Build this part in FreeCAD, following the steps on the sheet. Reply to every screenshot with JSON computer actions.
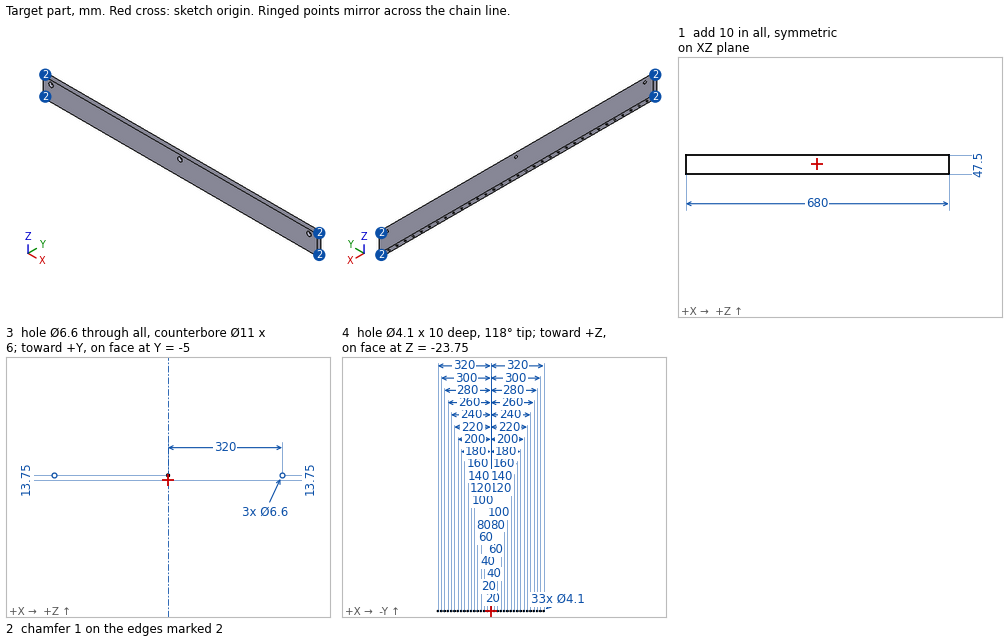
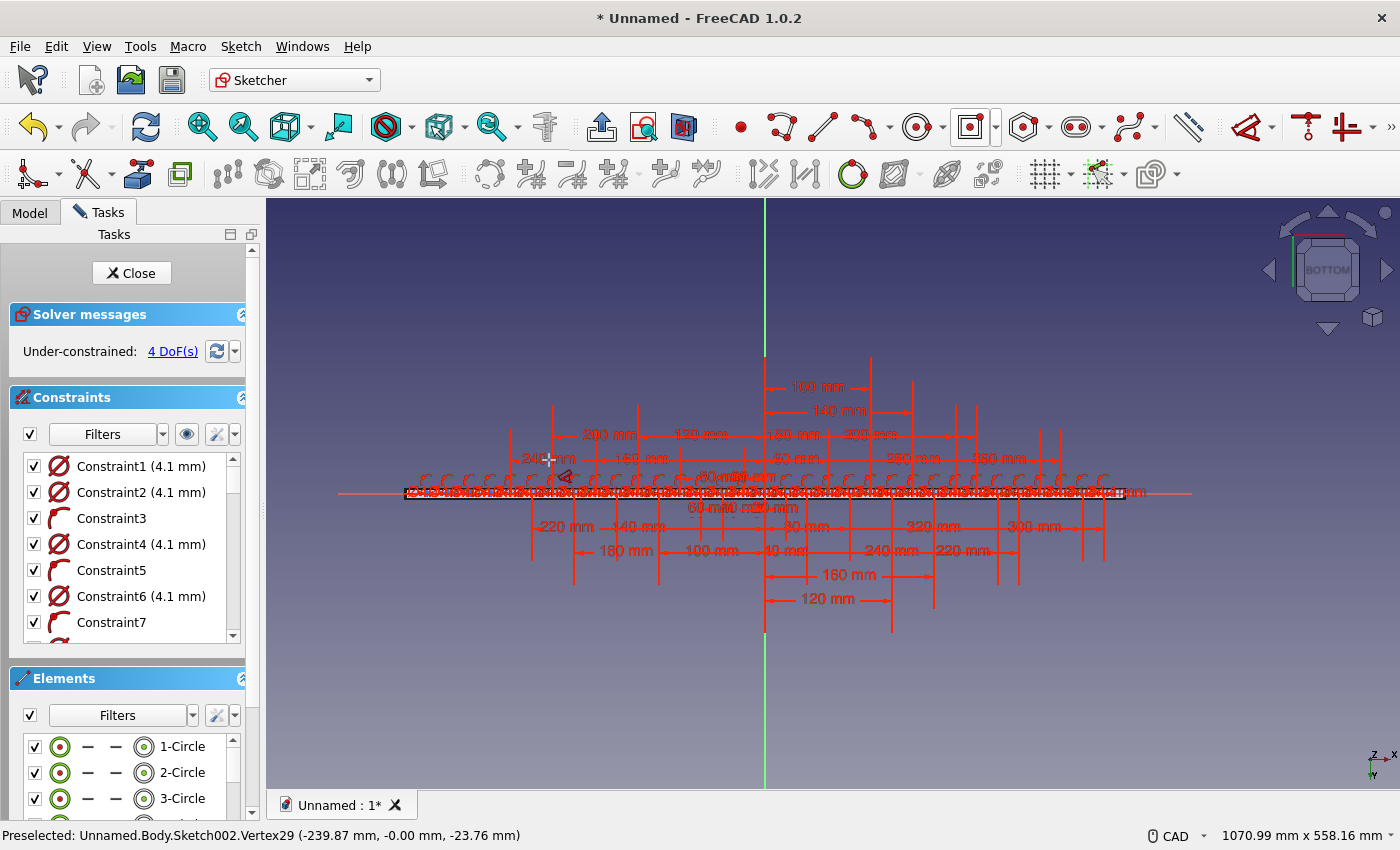
{"action": "left_click", "coordinate": [490, 494]}
{"action": "left_click", "coordinate": [531, 552]}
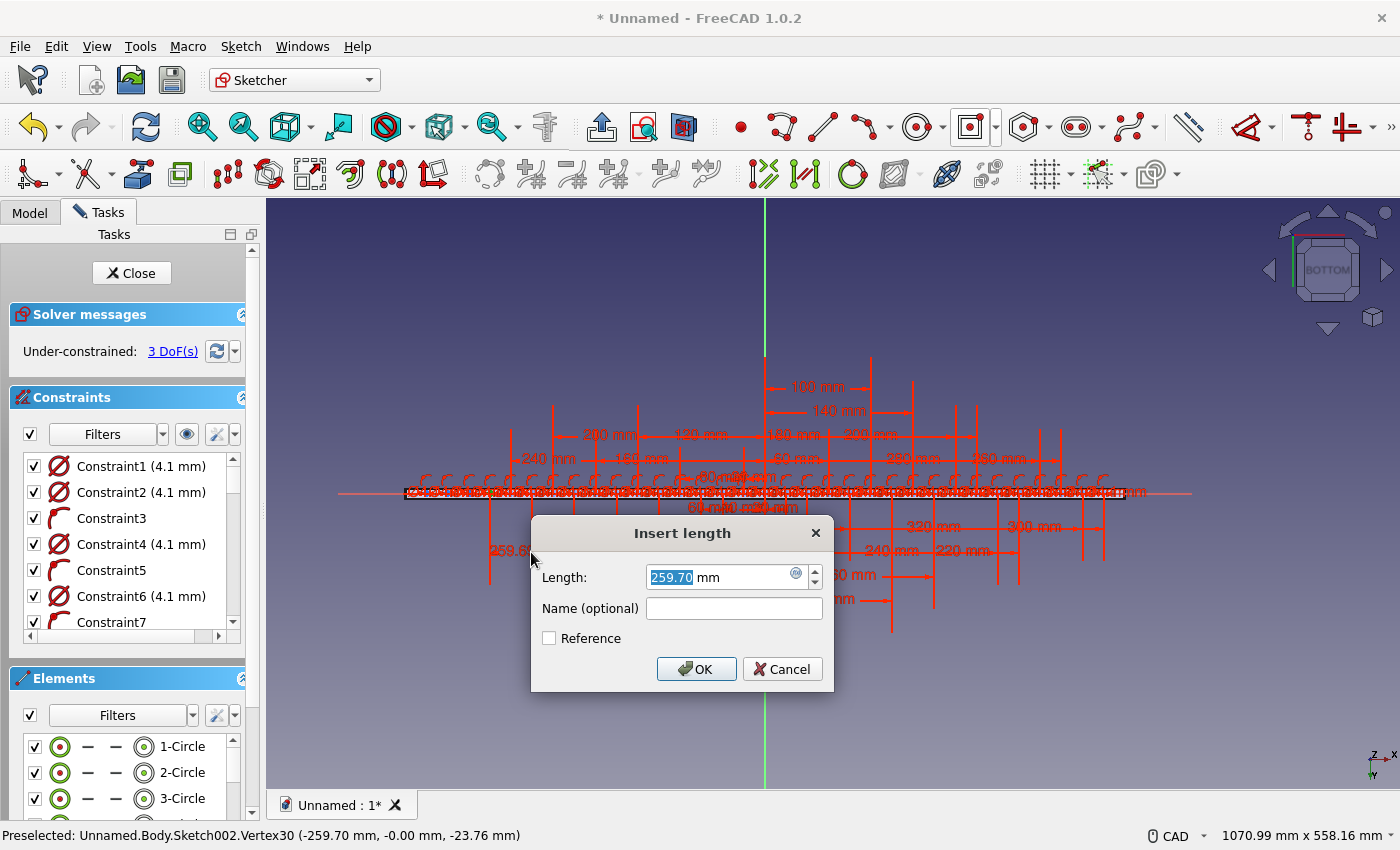
{"action": "type", "text": "260"}
{"action": "key", "text": "Return"}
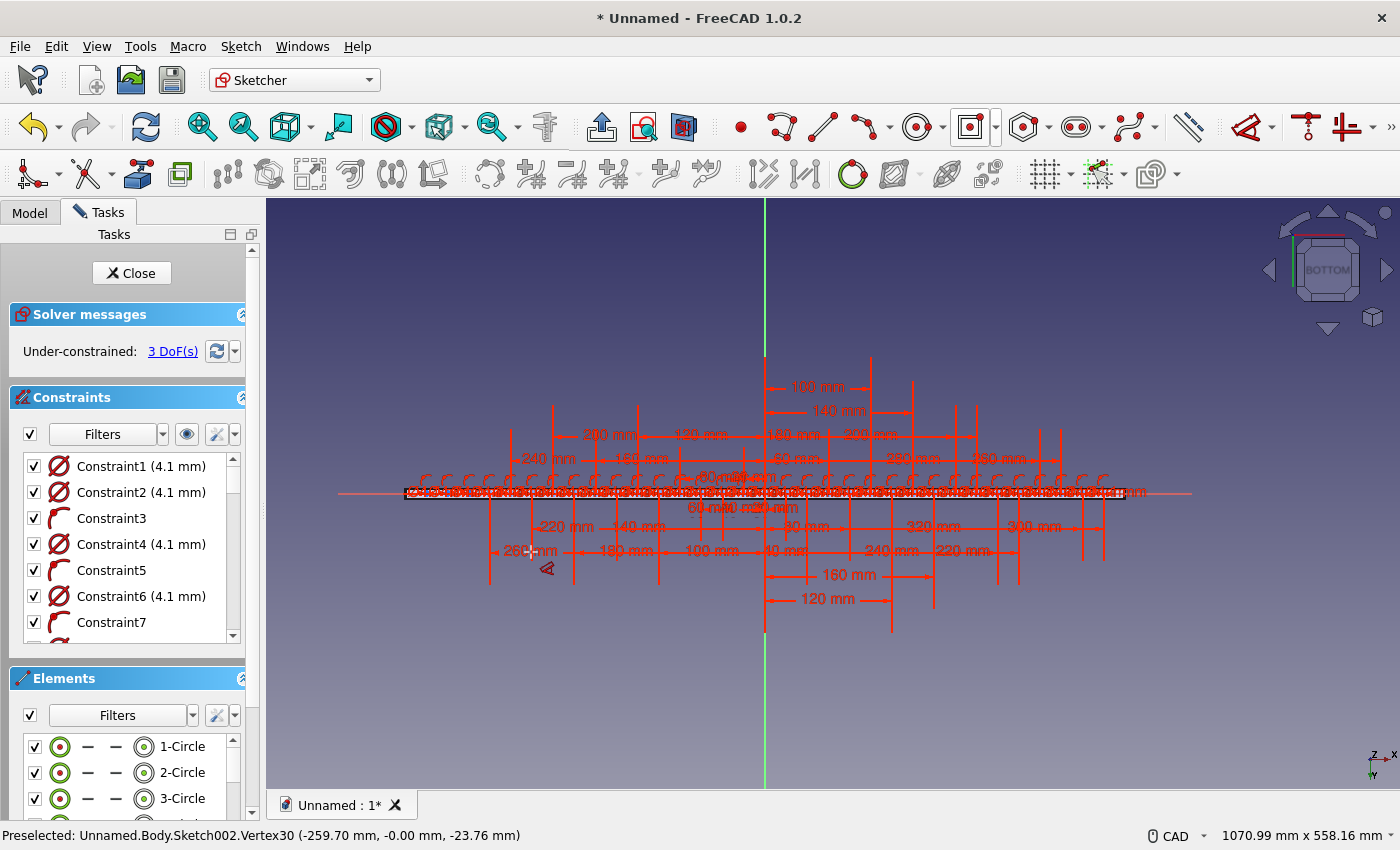
{"action": "left_click", "coordinate": [469, 494]}
{"action": "left_click", "coordinate": [513, 436]}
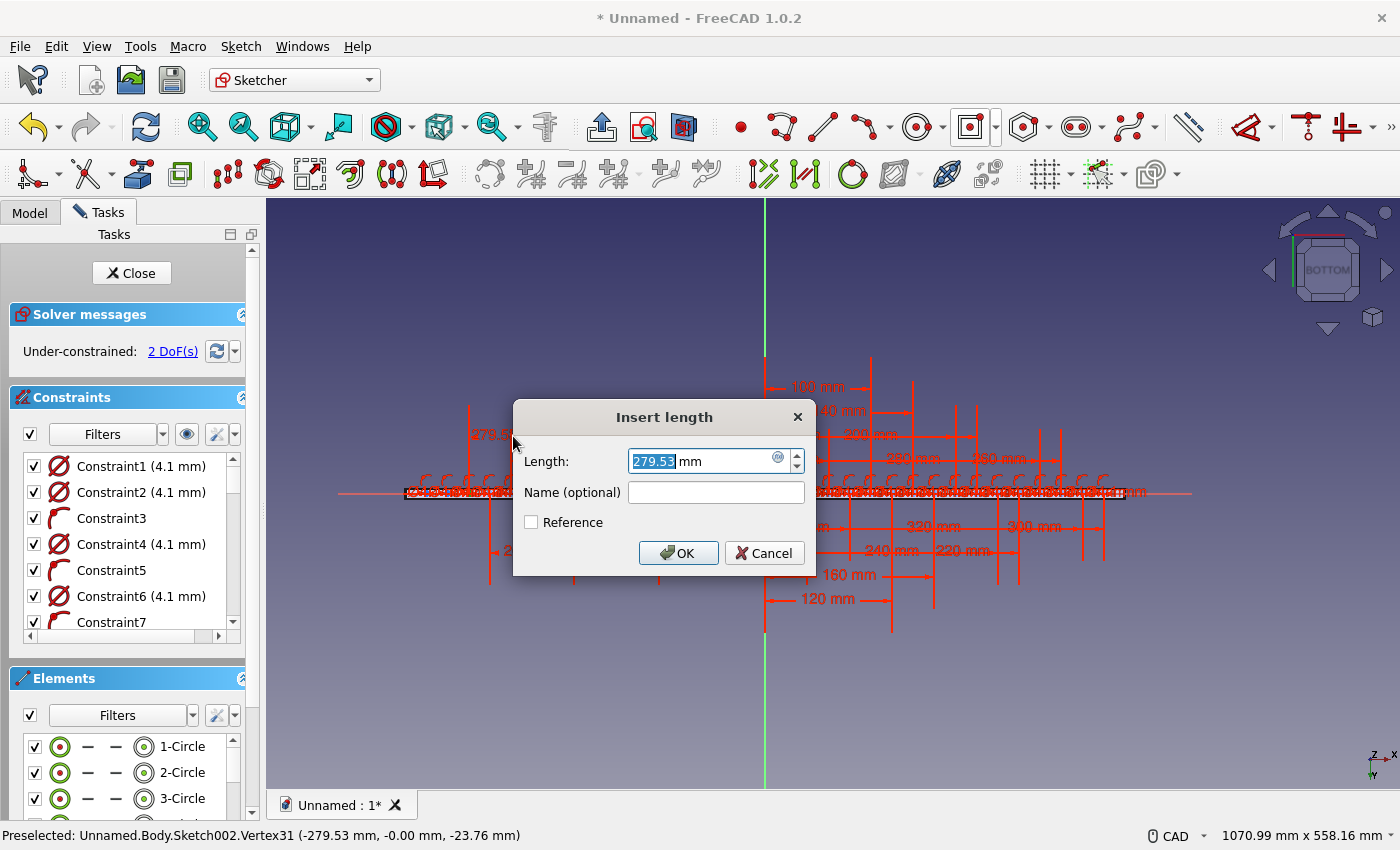
{"action": "type", "text": "280"}
{"action": "key", "text": "Return"}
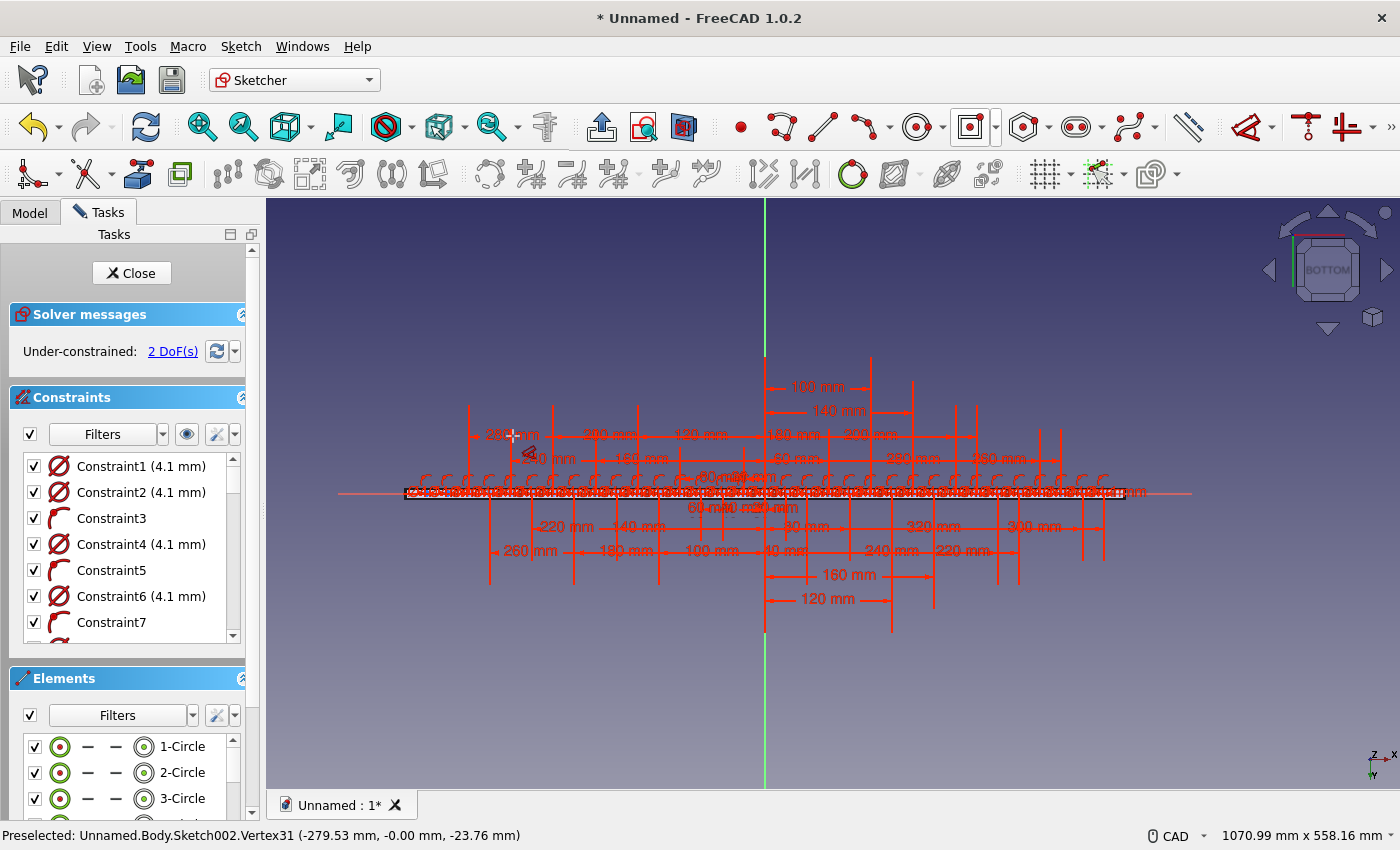
{"action": "left_click", "coordinate": [447, 494]}
{"action": "left_click", "coordinate": [495, 528]}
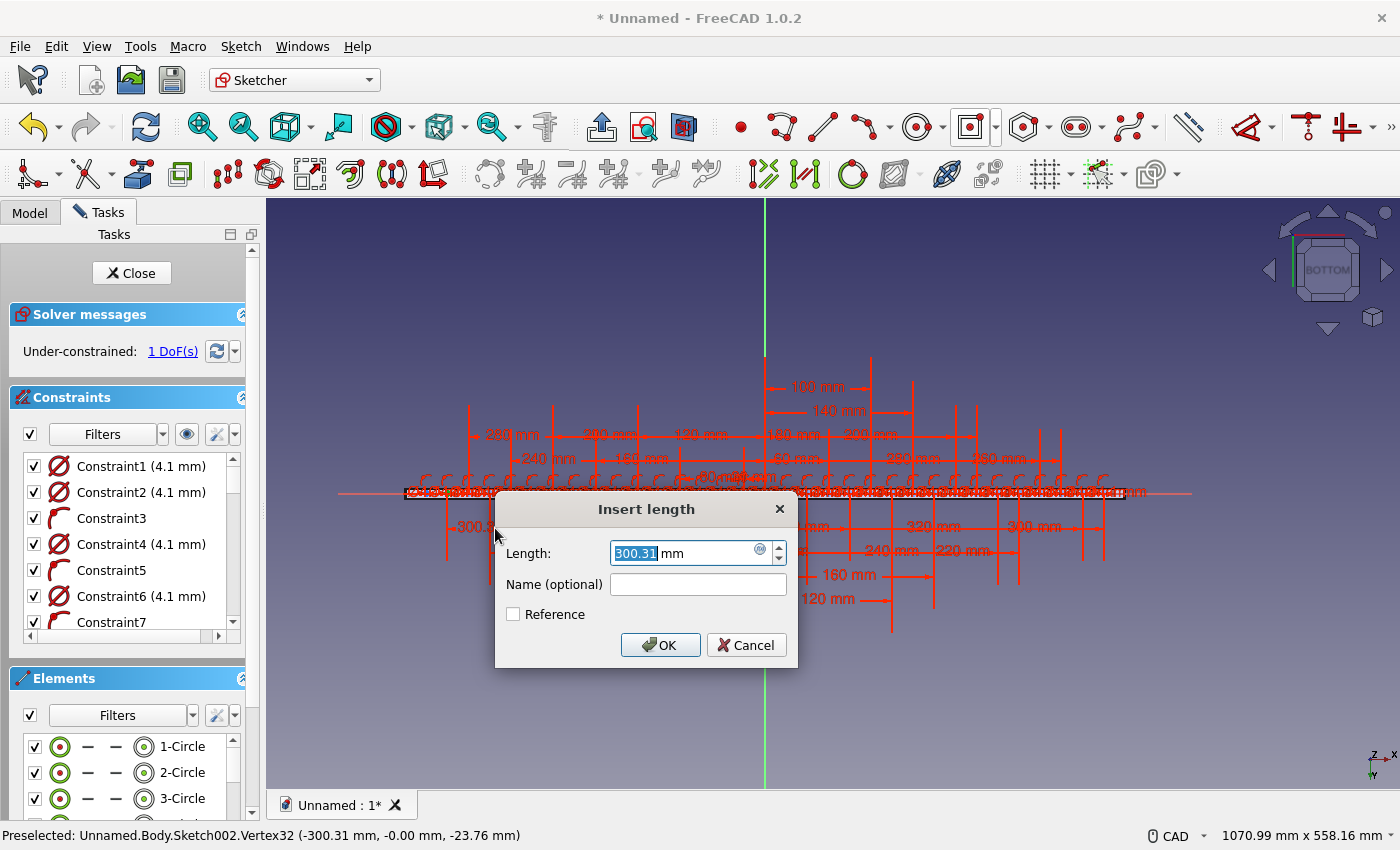
{"action": "type", "text": "300"}
{"action": "key", "text": "Return"}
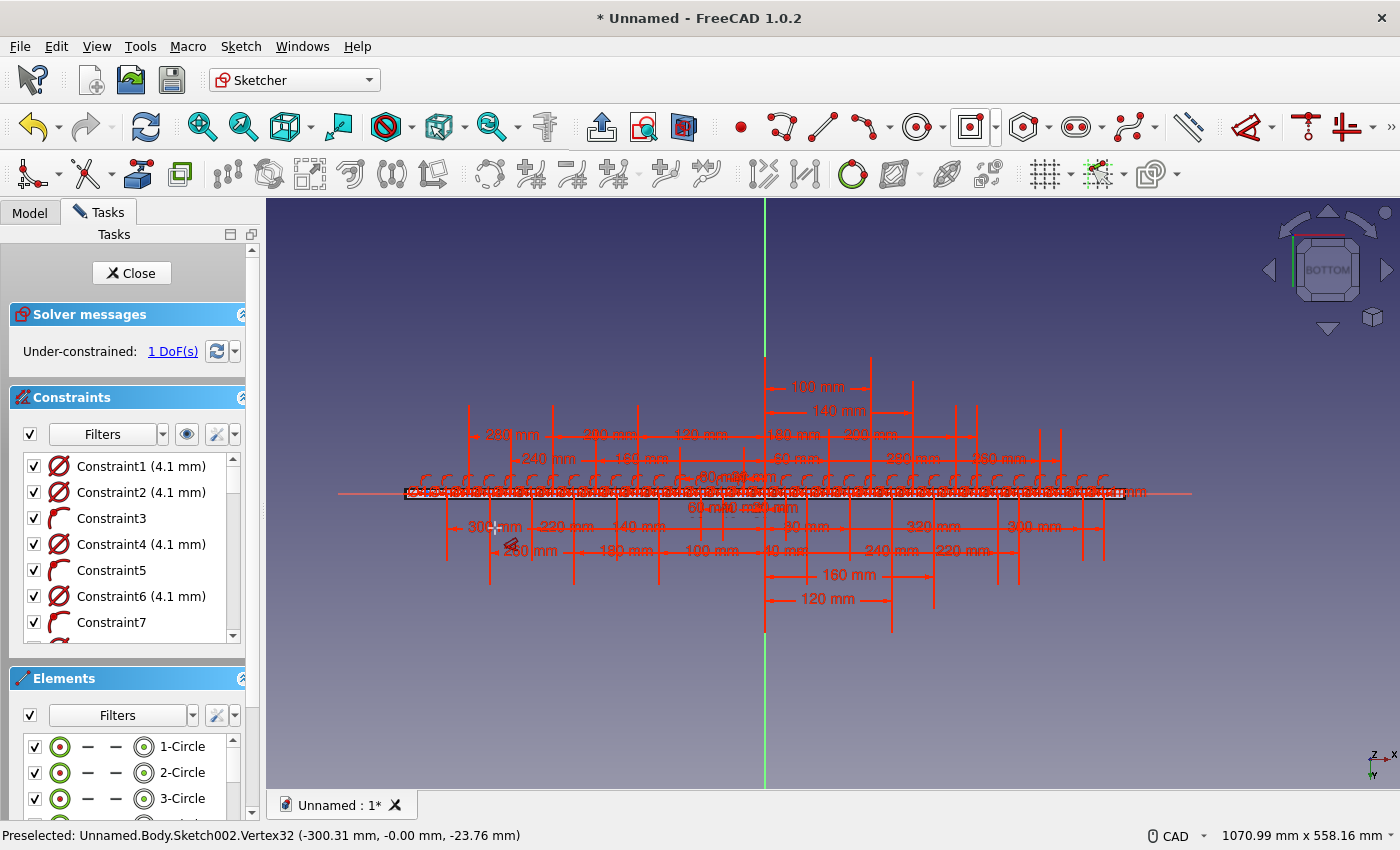
{"action": "left_click", "coordinate": [426, 494]}
{"action": "left_click", "coordinate": [477, 460]}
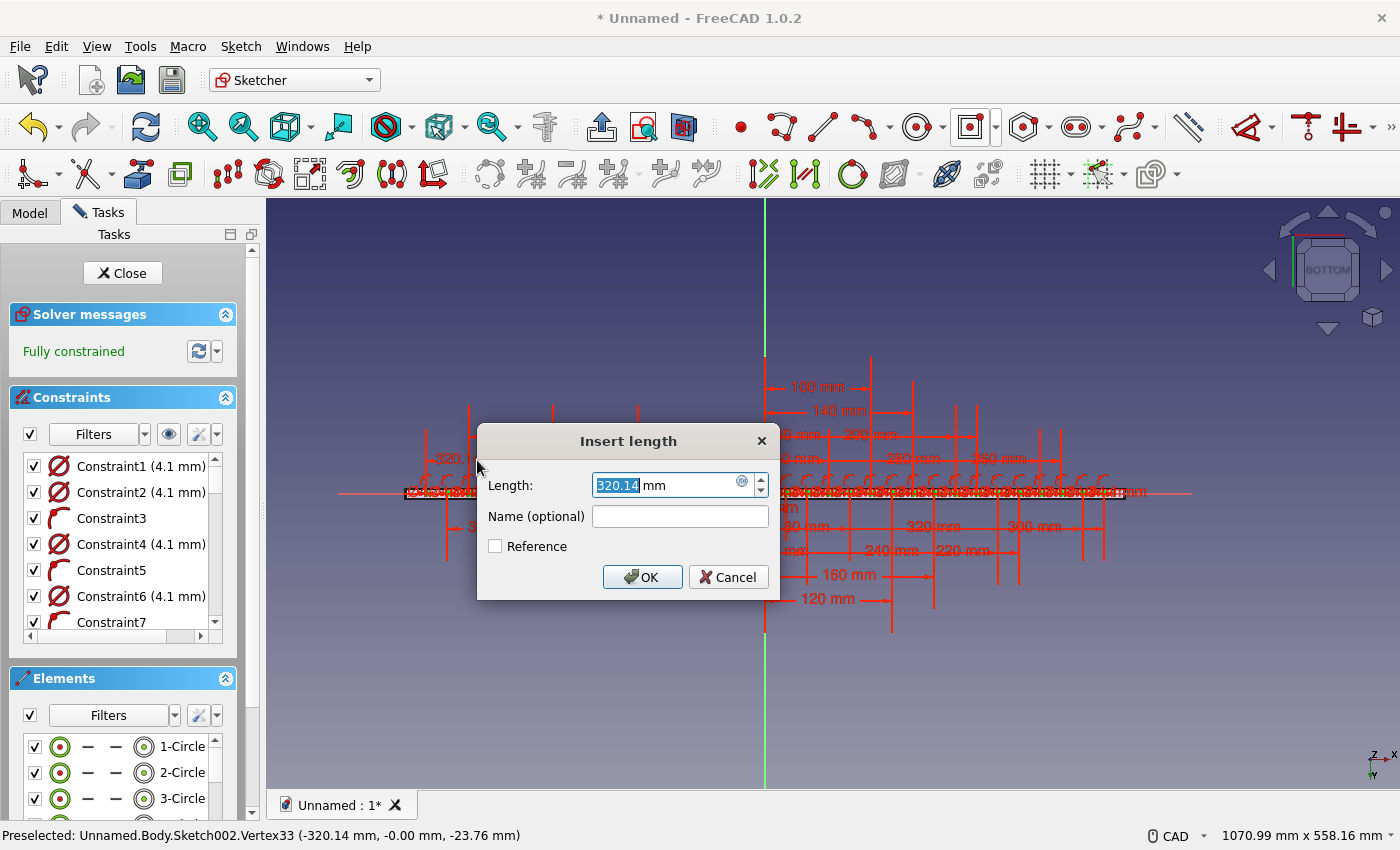
{"action": "type", "text": "320"}
{"action": "key", "text": "Return"}
{"action": "key", "text": "Escape"}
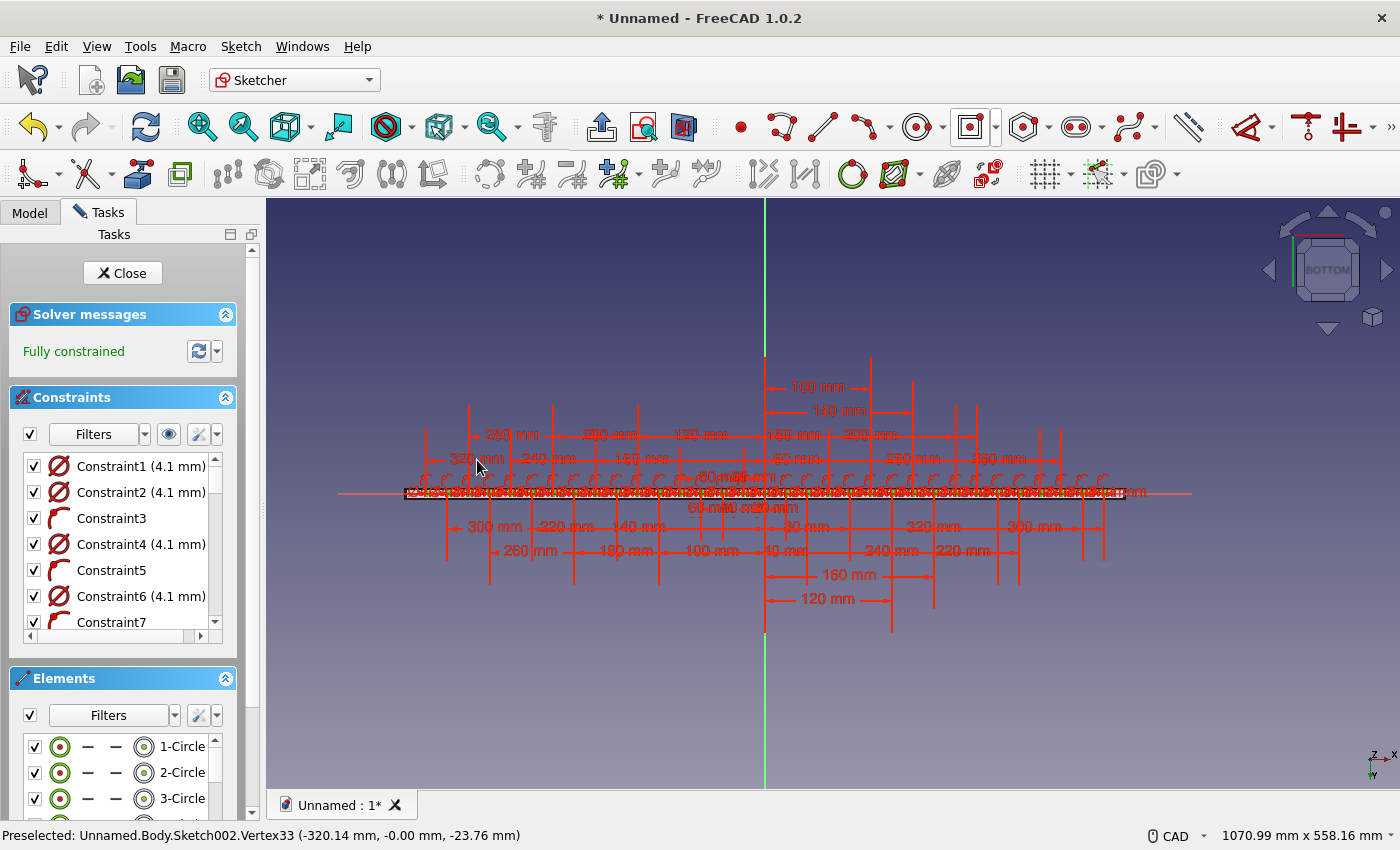
{"action": "left_click", "coordinate": [123, 273]}